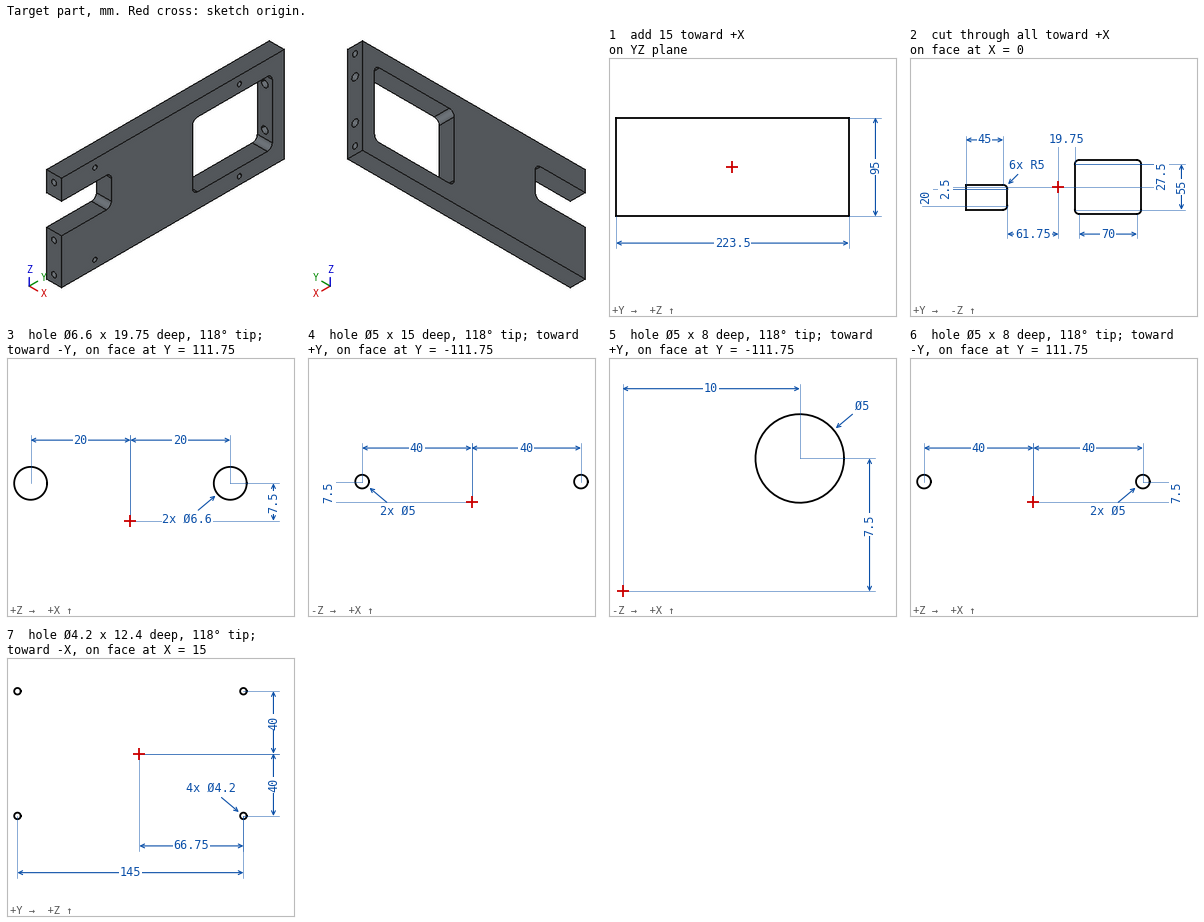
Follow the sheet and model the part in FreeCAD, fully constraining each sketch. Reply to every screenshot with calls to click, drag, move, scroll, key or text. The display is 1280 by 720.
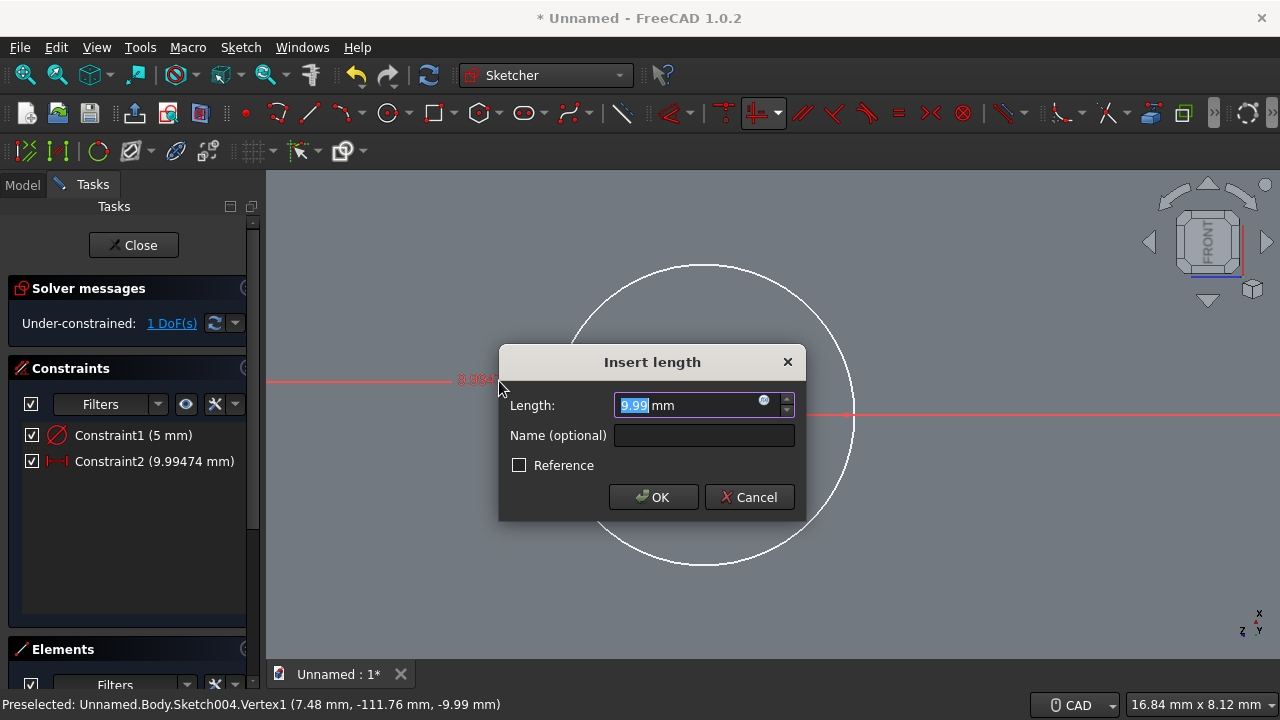
text(10)
key(Return)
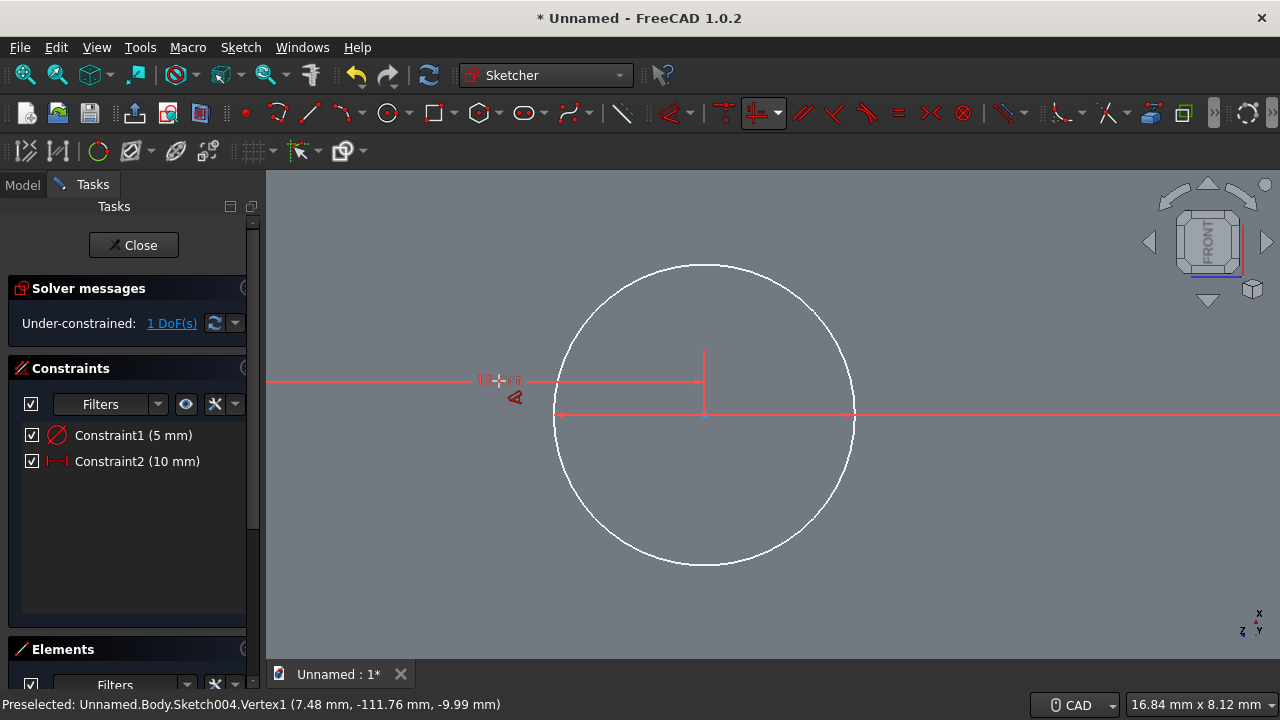
click(704, 415)
click(738, 523)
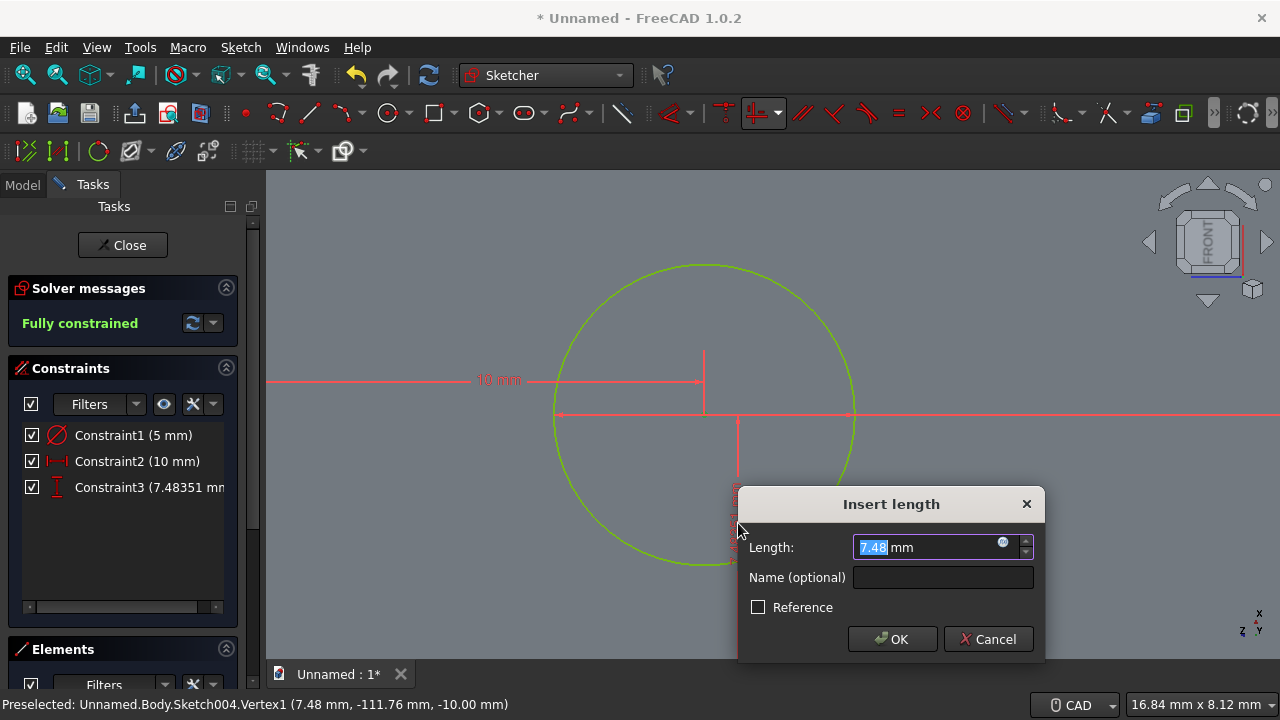
text(7.5)
key(Return)
key(Escape)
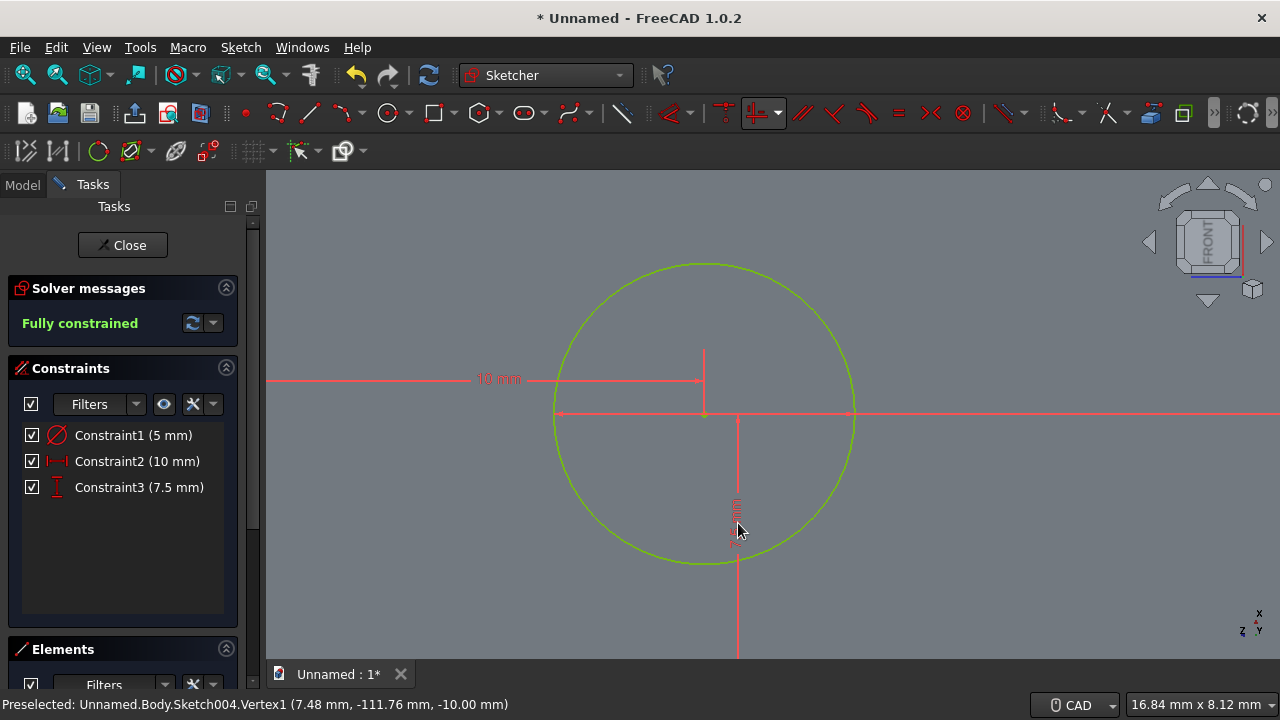
click(123, 245)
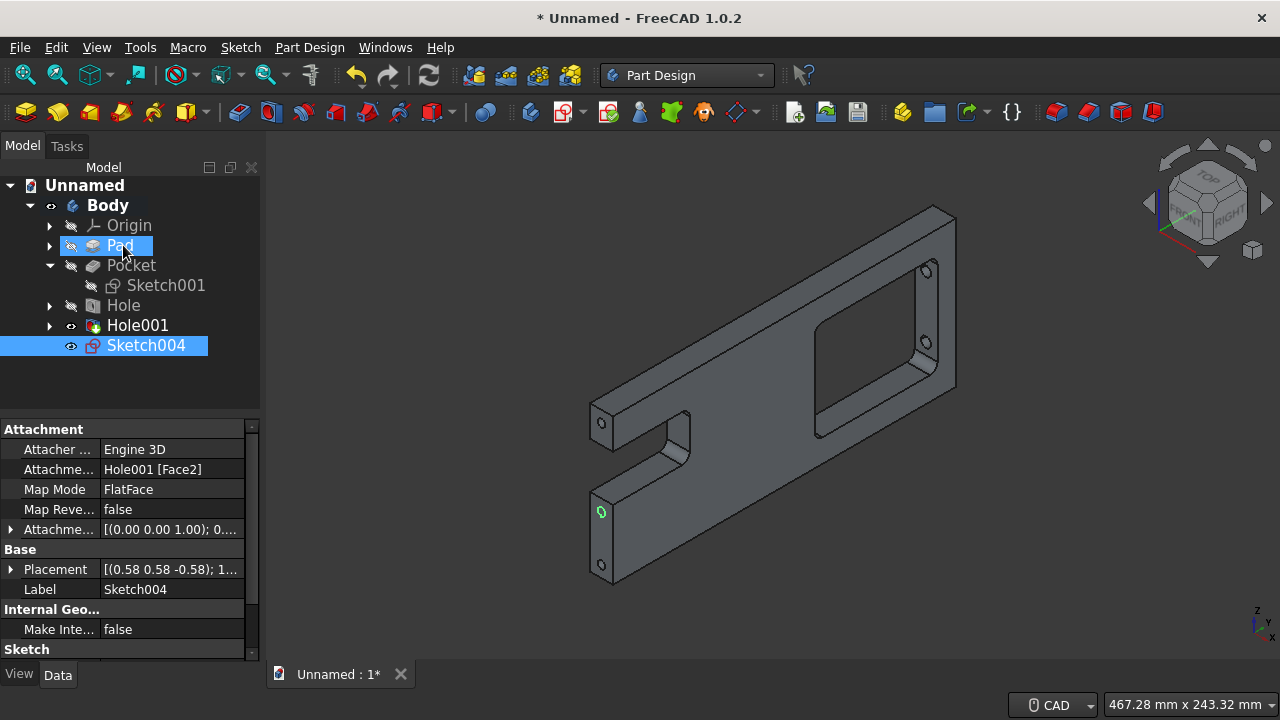
click(272, 112)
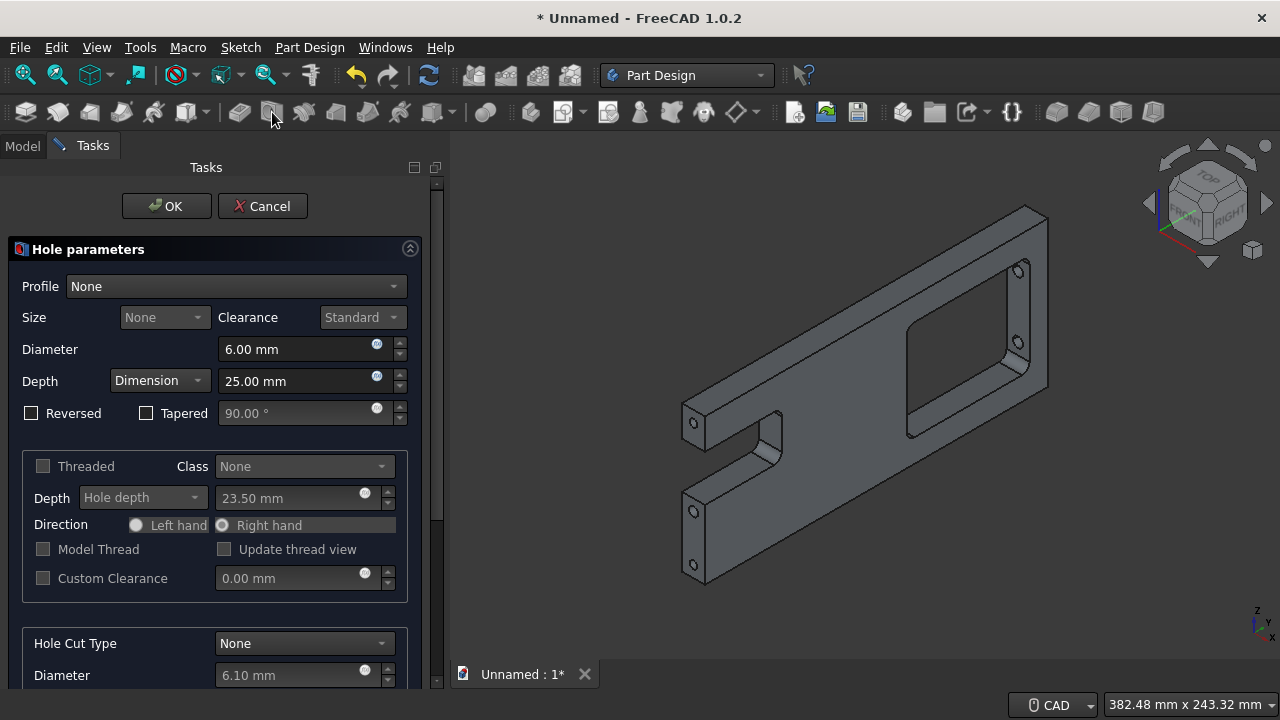
triple_click(305, 349)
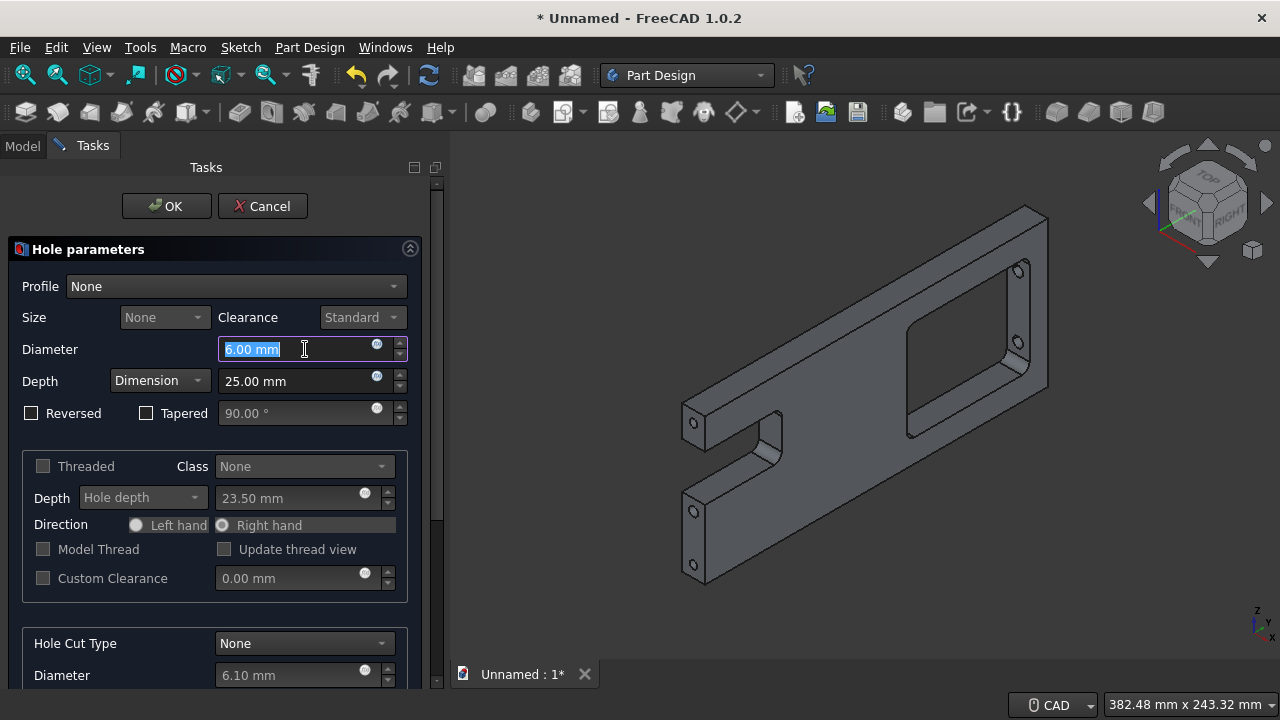
text(5)
key(Tab)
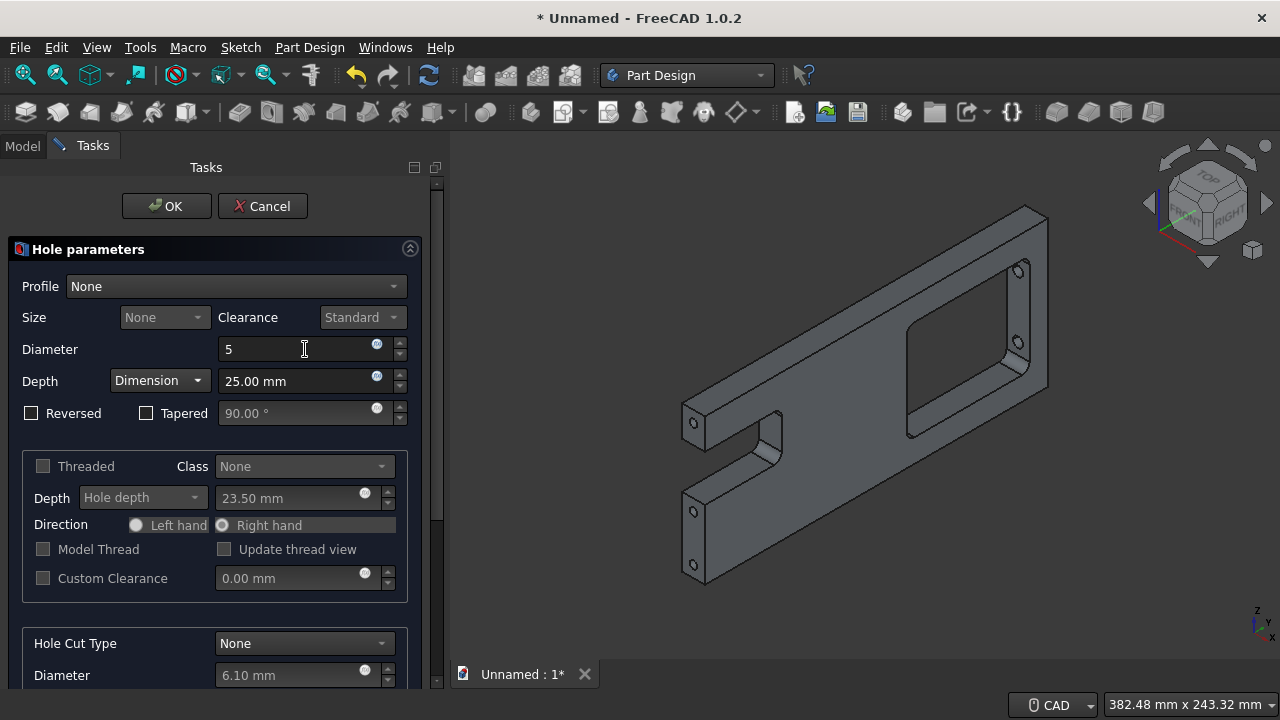
triple_click(305, 381)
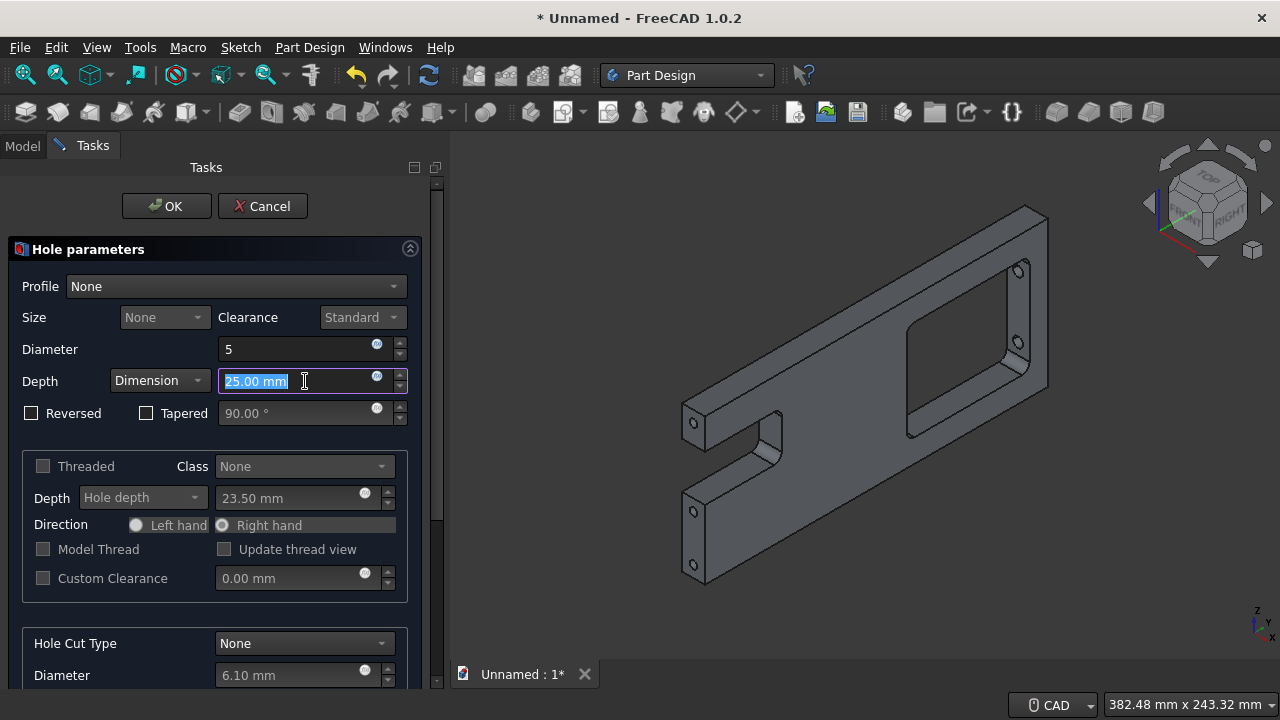
text(8)
key(Tab)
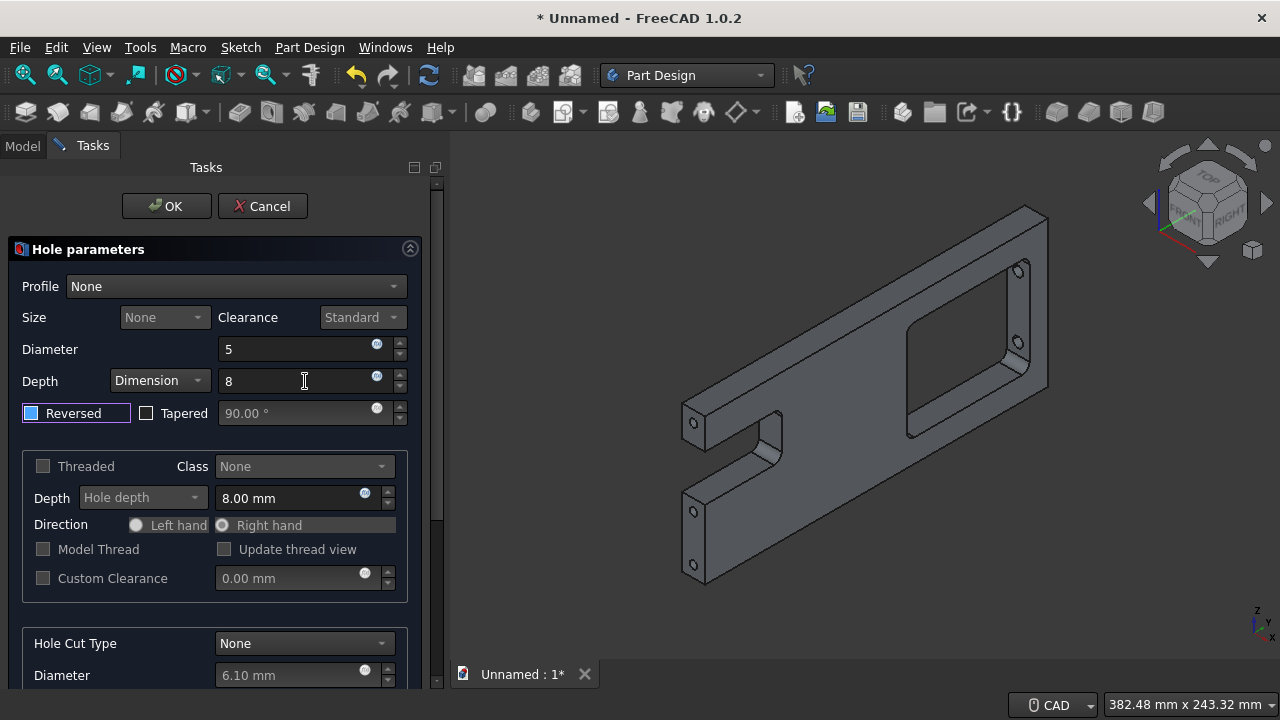
click(167, 206)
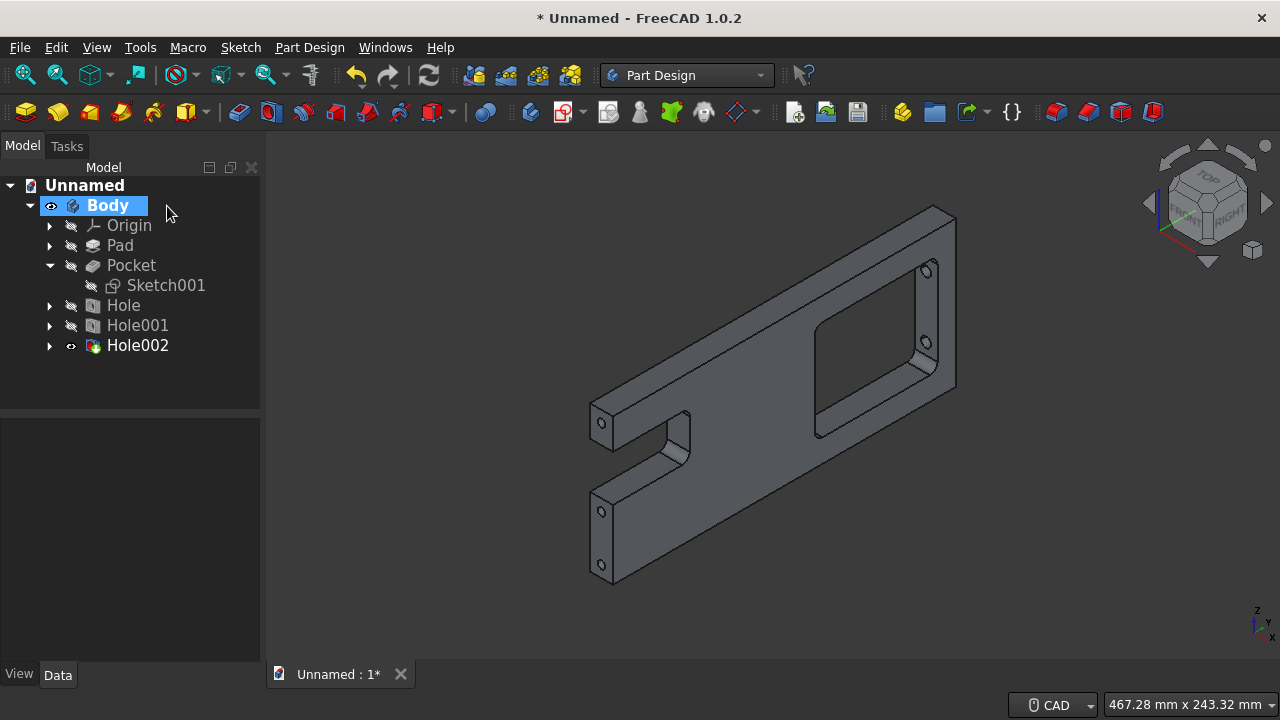
key(4)